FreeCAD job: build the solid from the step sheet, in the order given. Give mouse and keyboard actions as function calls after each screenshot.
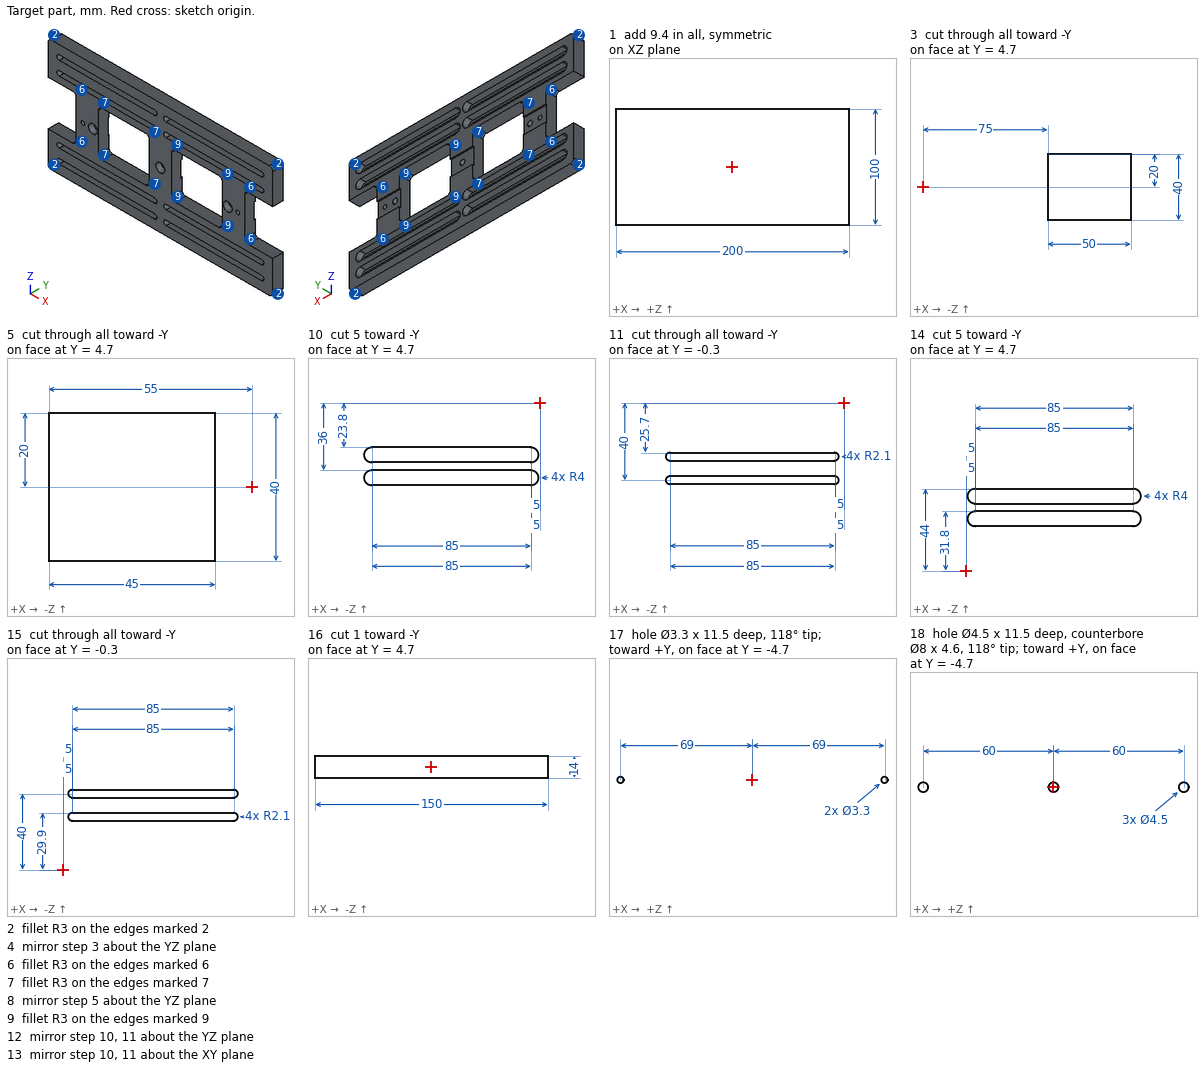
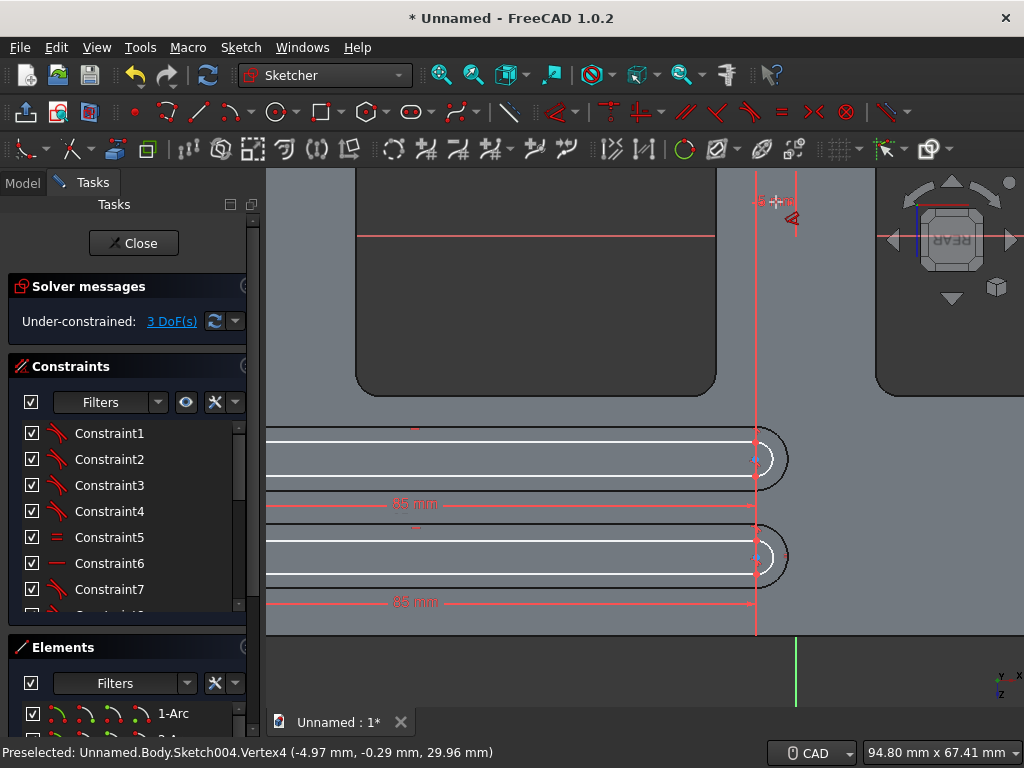
click(756, 574)
click(776, 608)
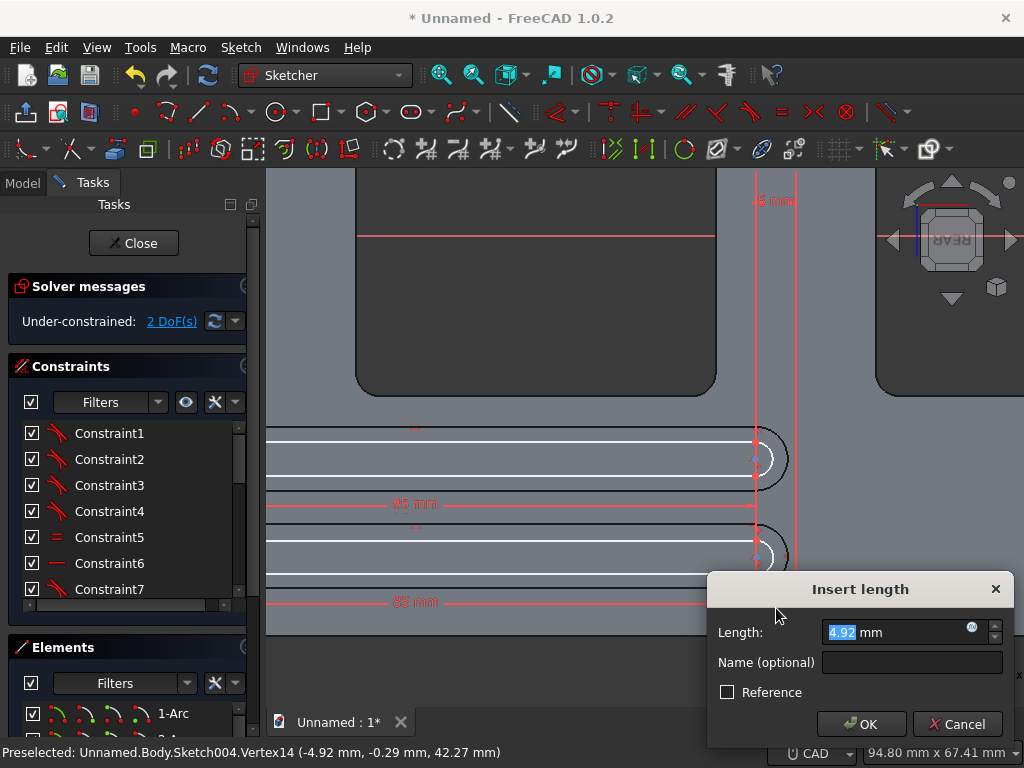
text(5)
key(Return)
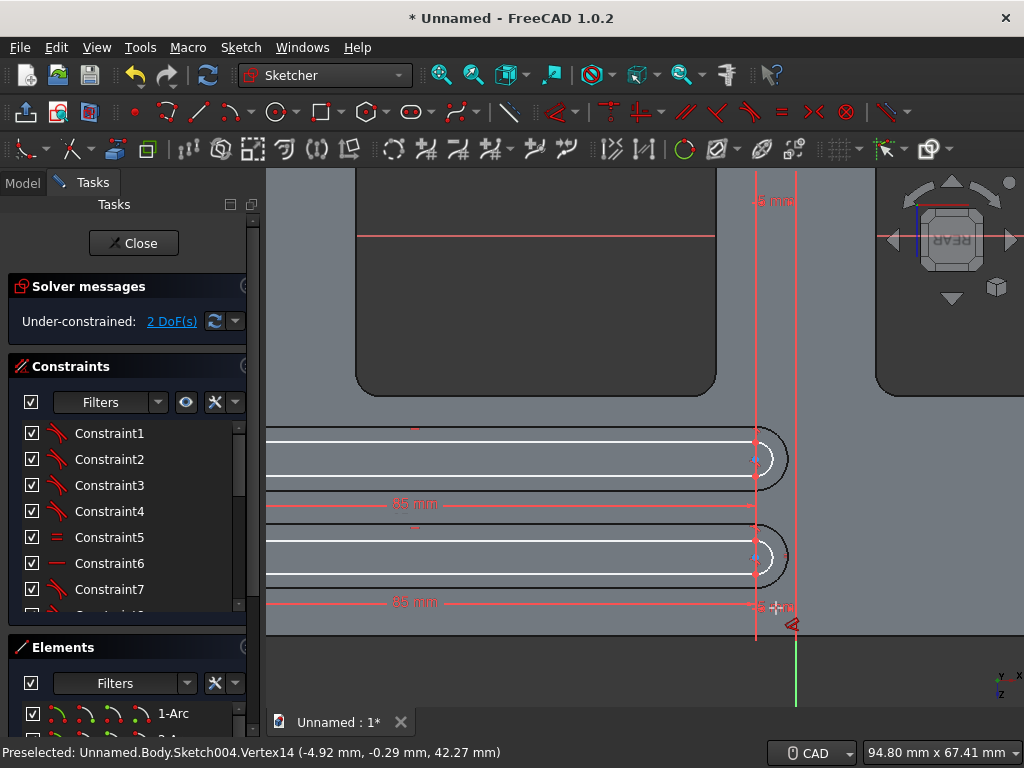
scroll(758, 477, down, 3)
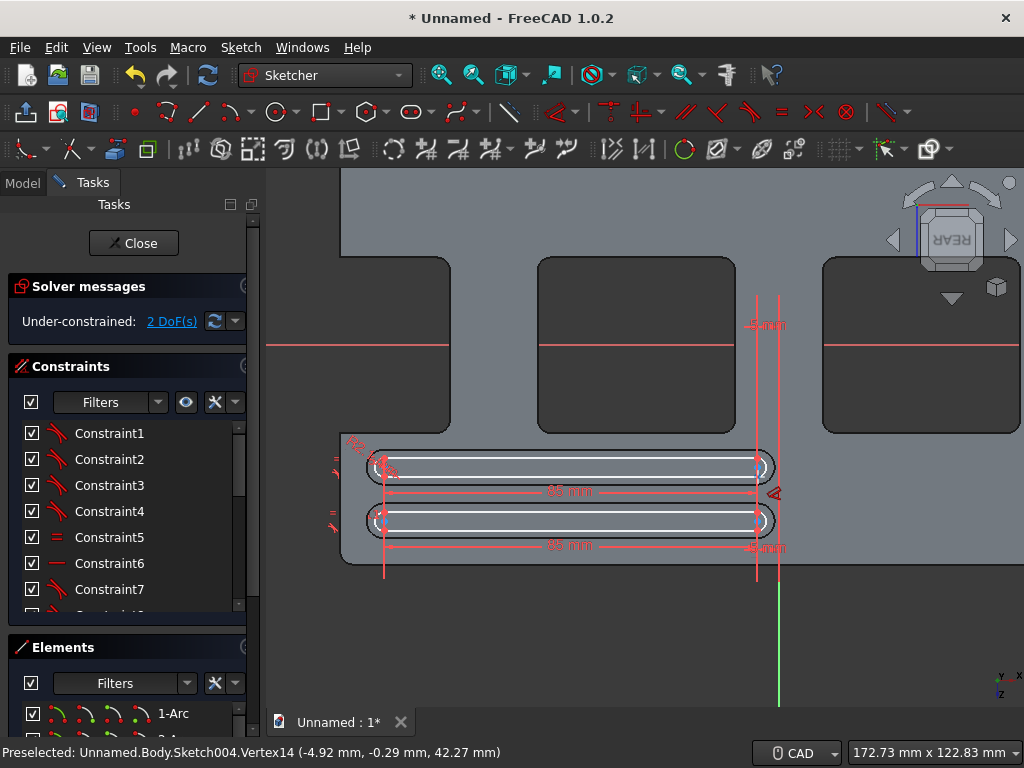
scroll(384, 522, up, 2)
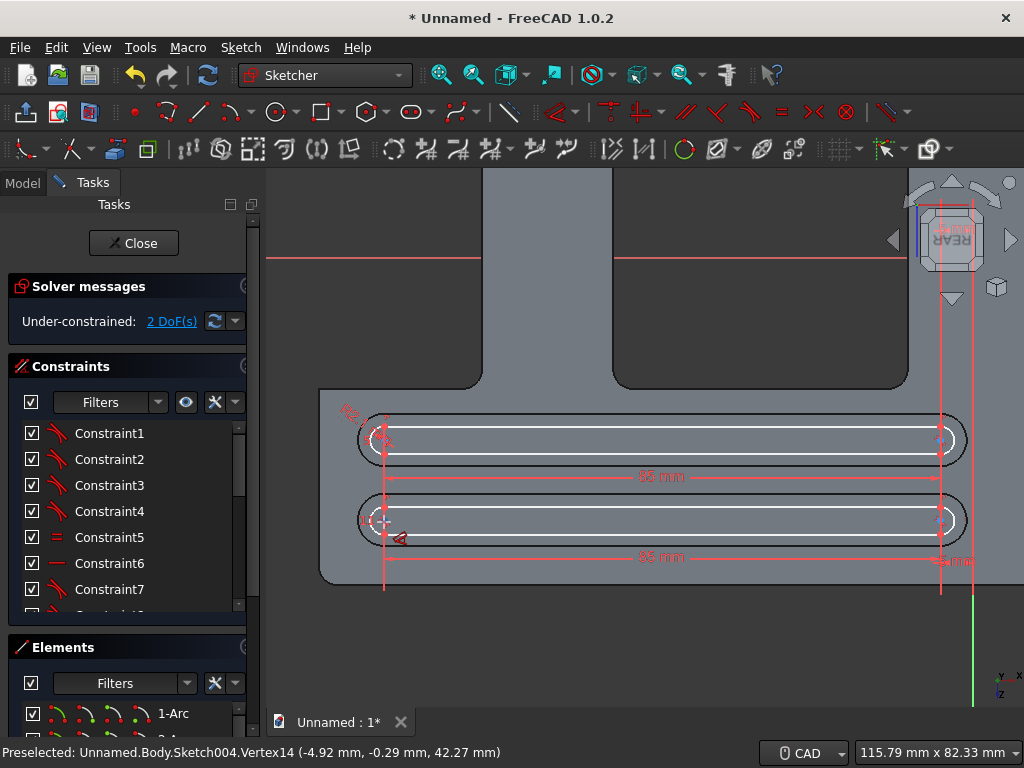
click(384, 521)
click(350, 389)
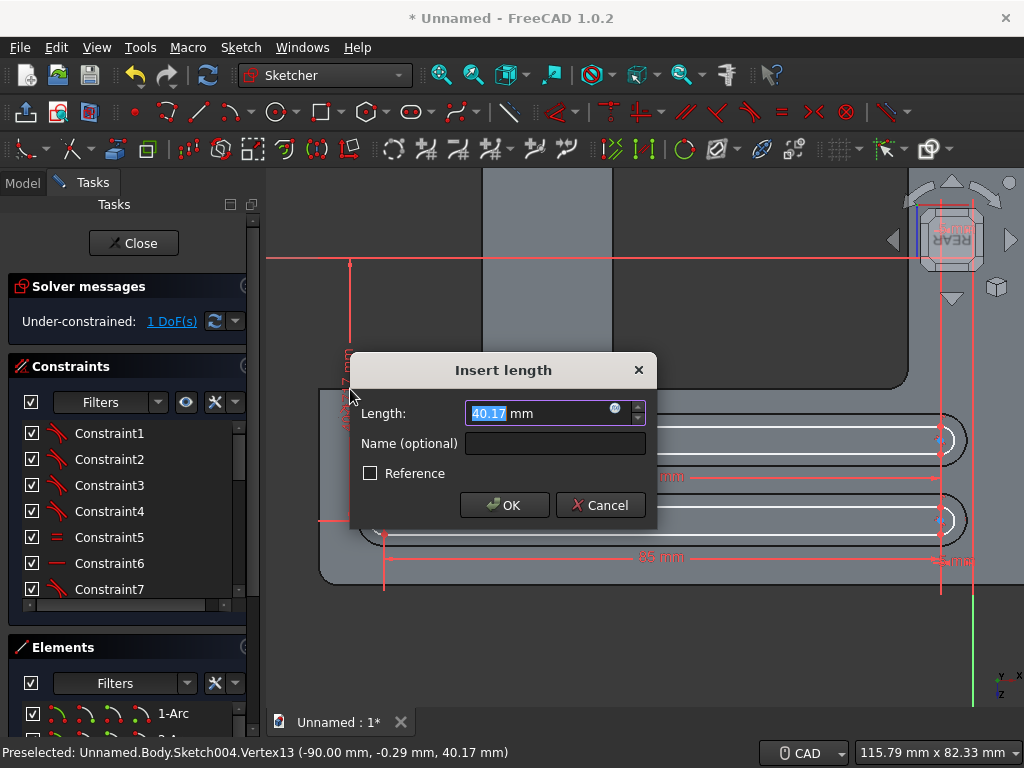
text(40)
key(Return)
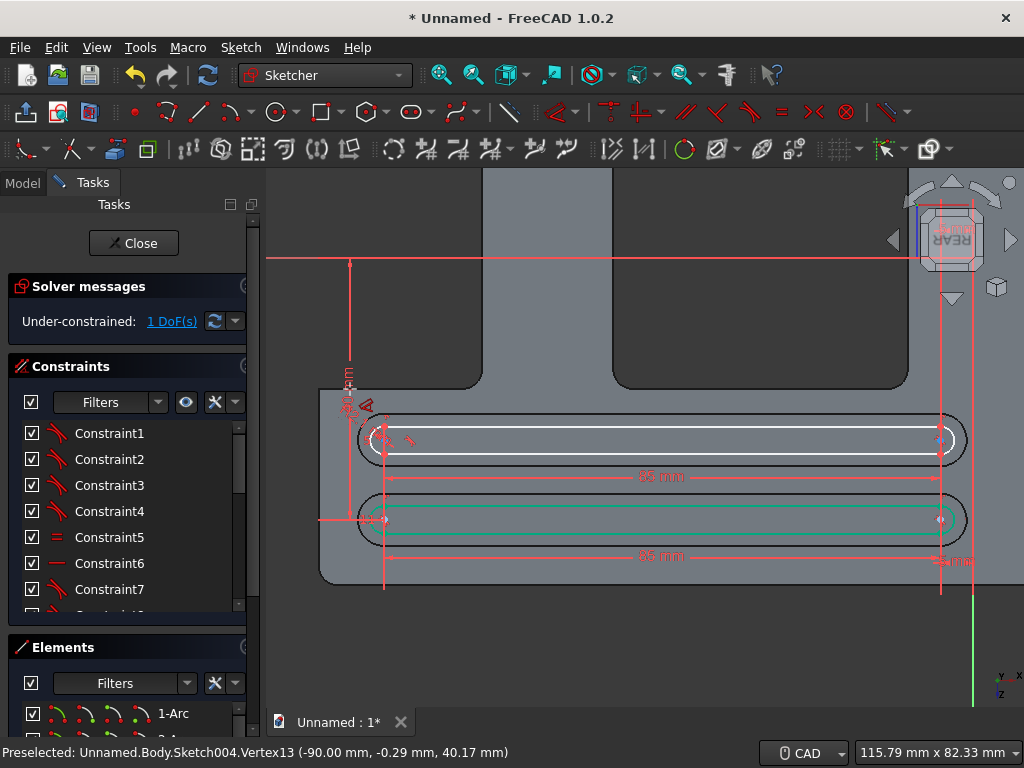
click(384, 427)
click(350, 342)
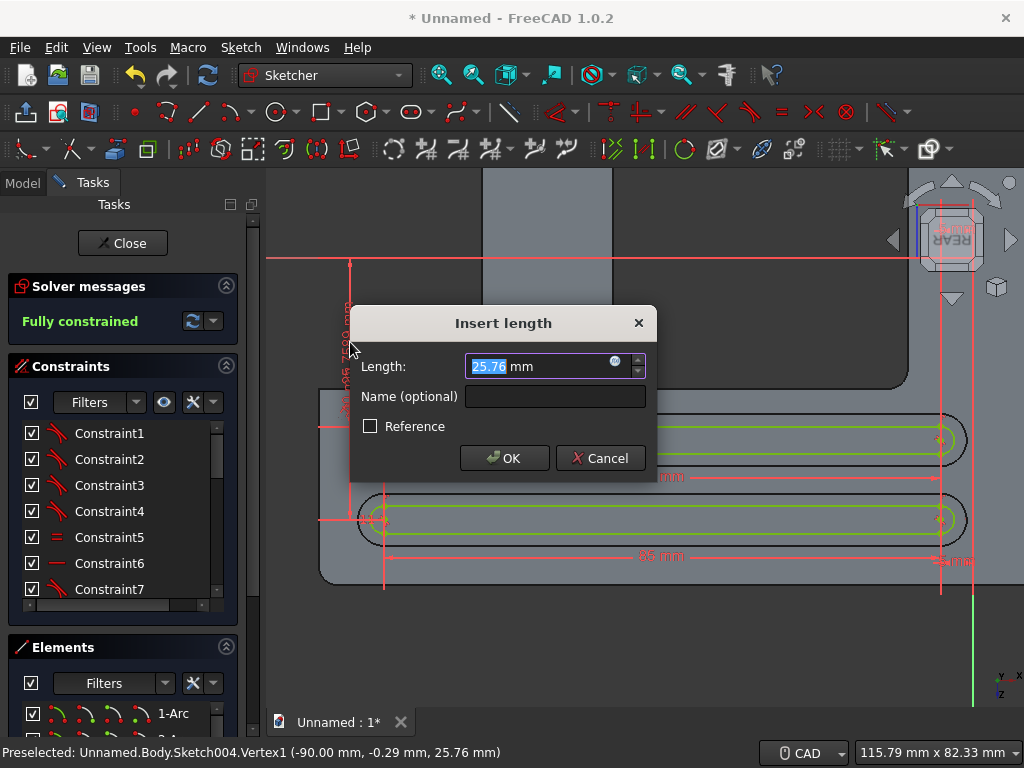
text(25.7)
key(Return)
key(Escape)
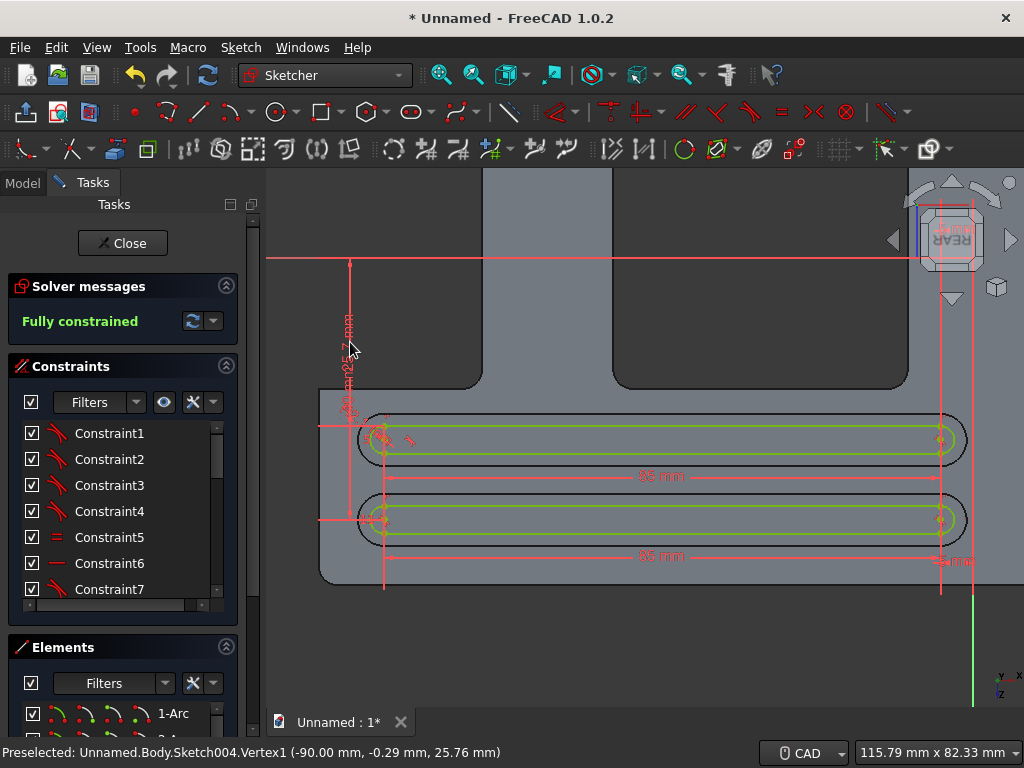
click(123, 243)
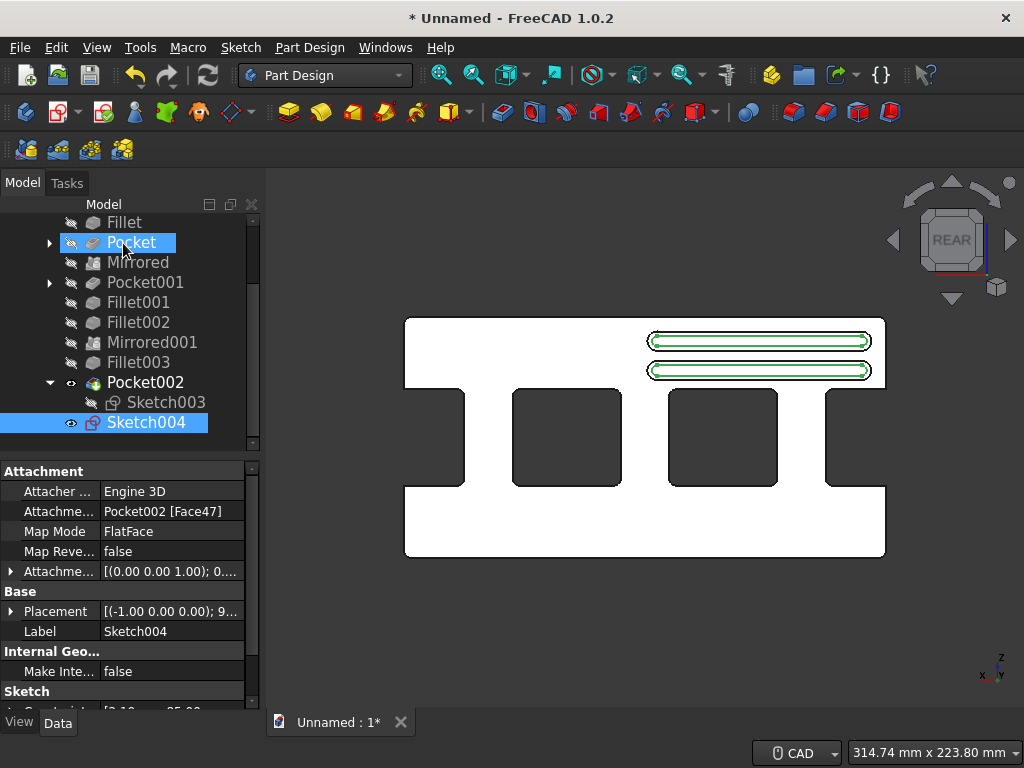
click(504, 112)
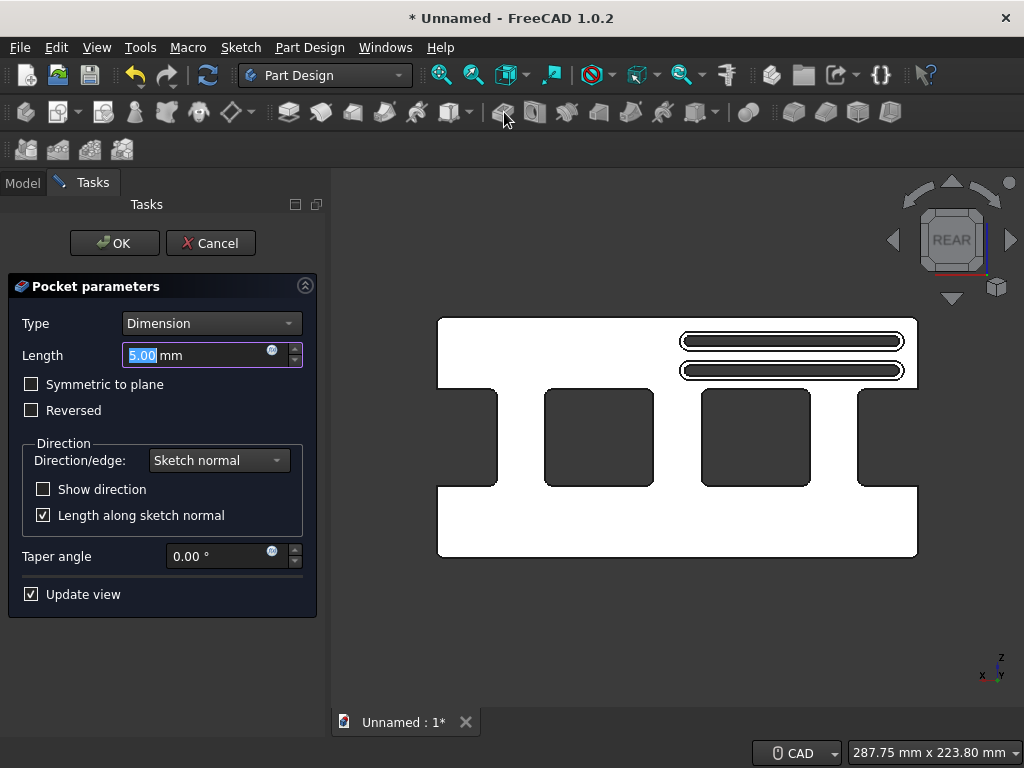
click(212, 324)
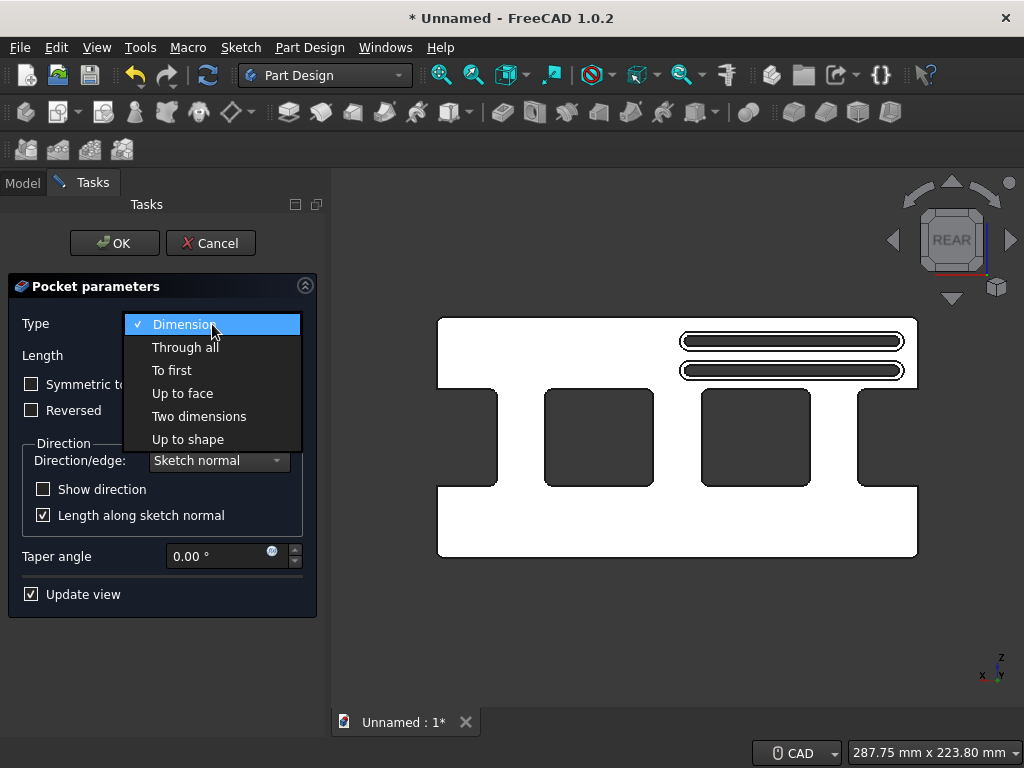
click(212, 348)